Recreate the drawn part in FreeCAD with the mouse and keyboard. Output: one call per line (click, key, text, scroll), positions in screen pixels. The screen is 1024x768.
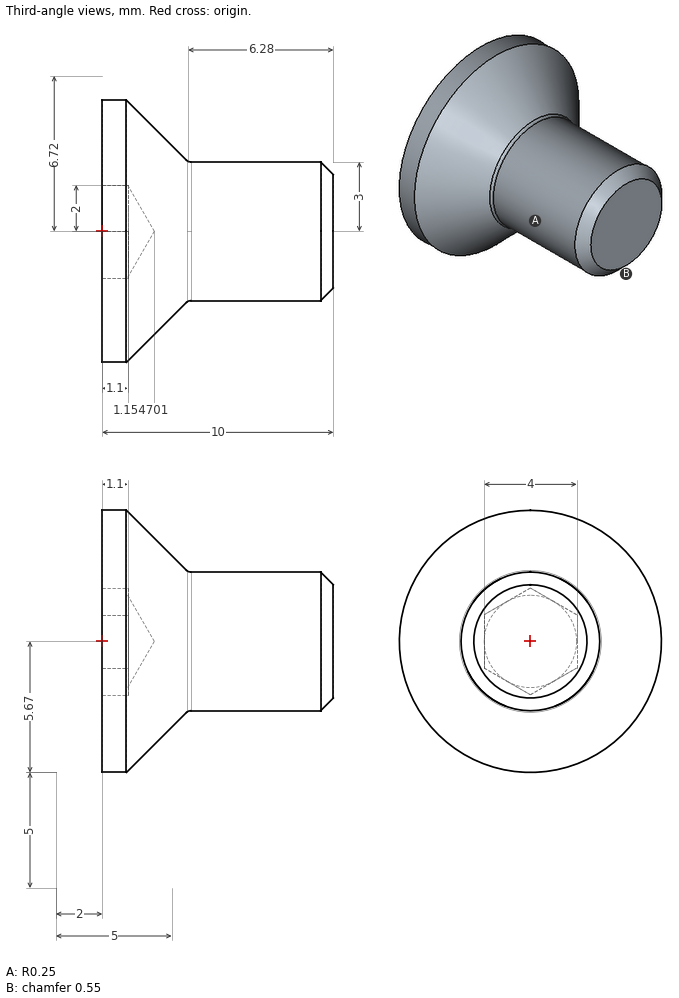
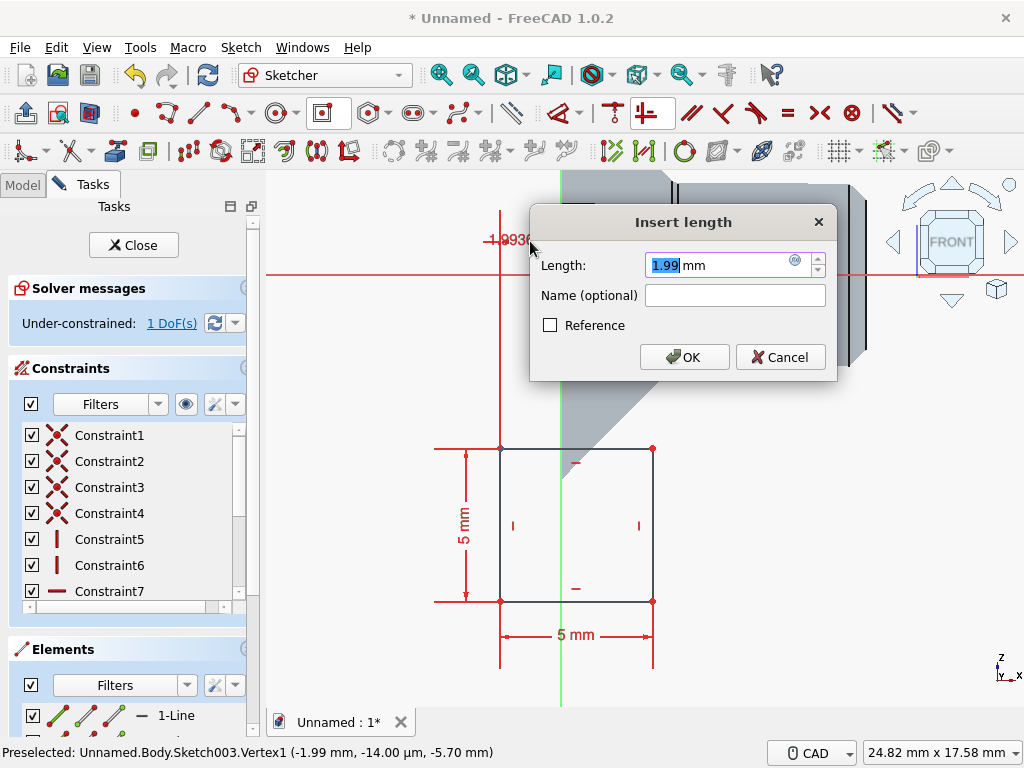
text(2)
key(Return)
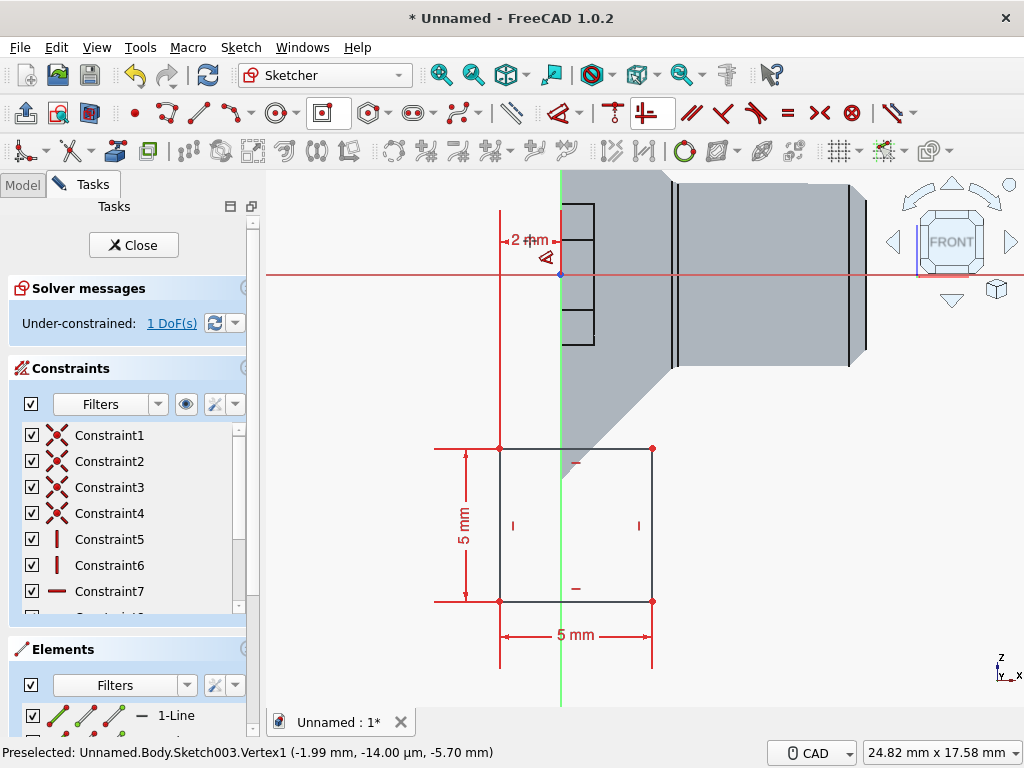
click(500, 449)
click(466, 362)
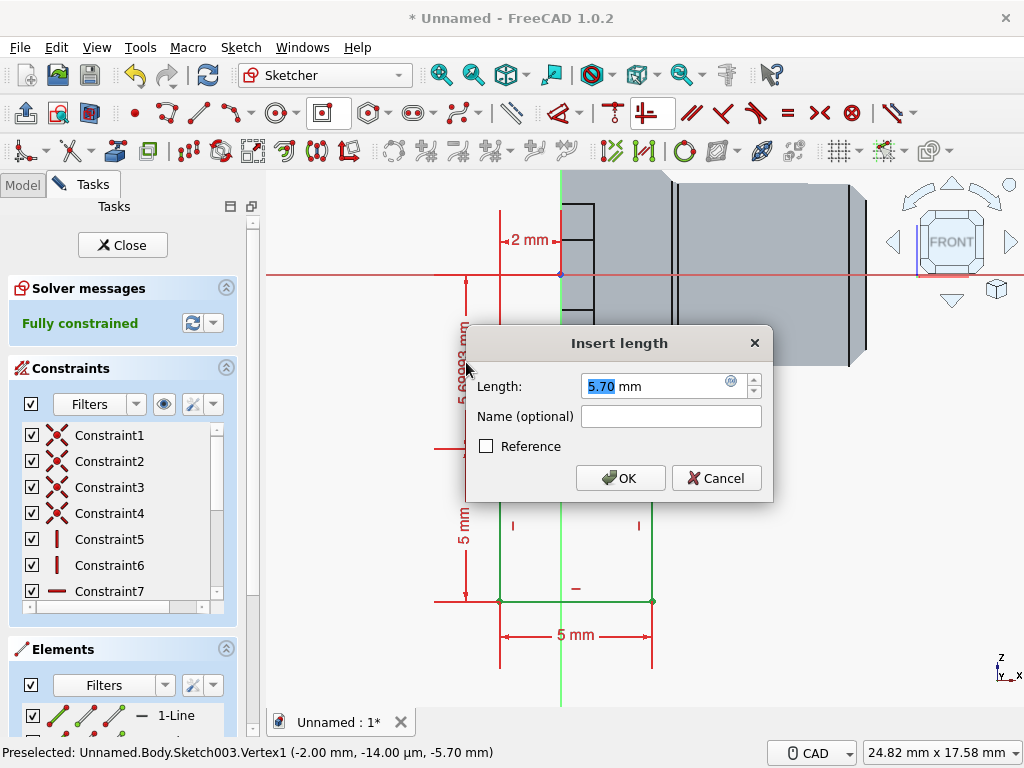
text(5.67)
key(Return)
key(Escape)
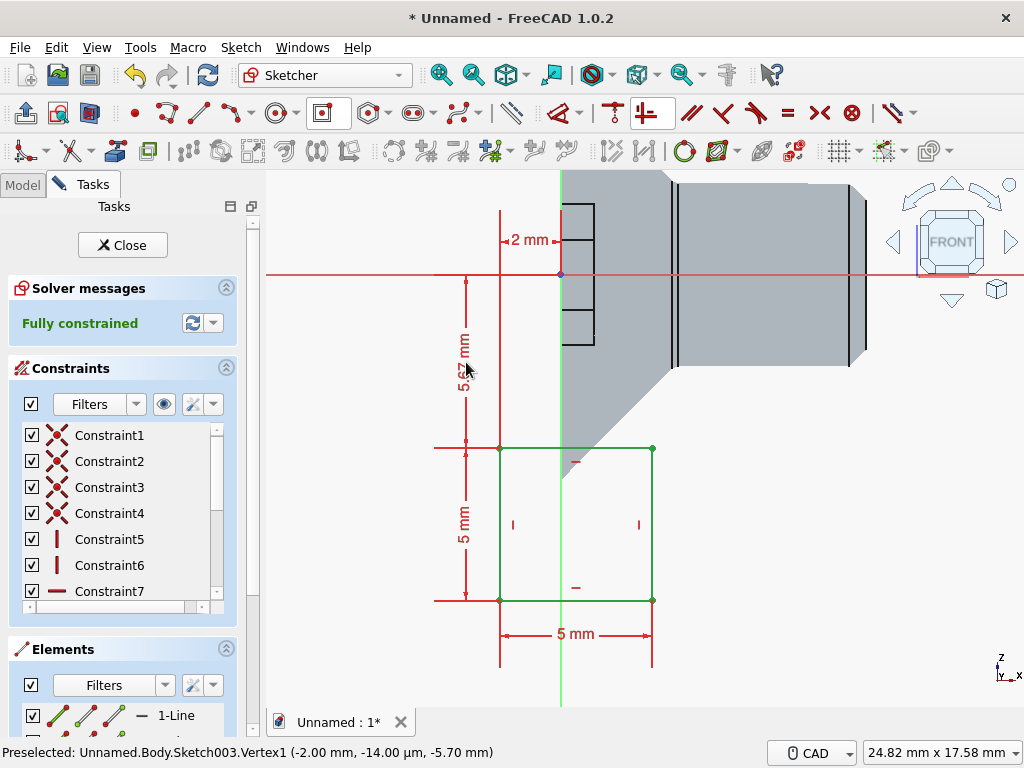
click(123, 245)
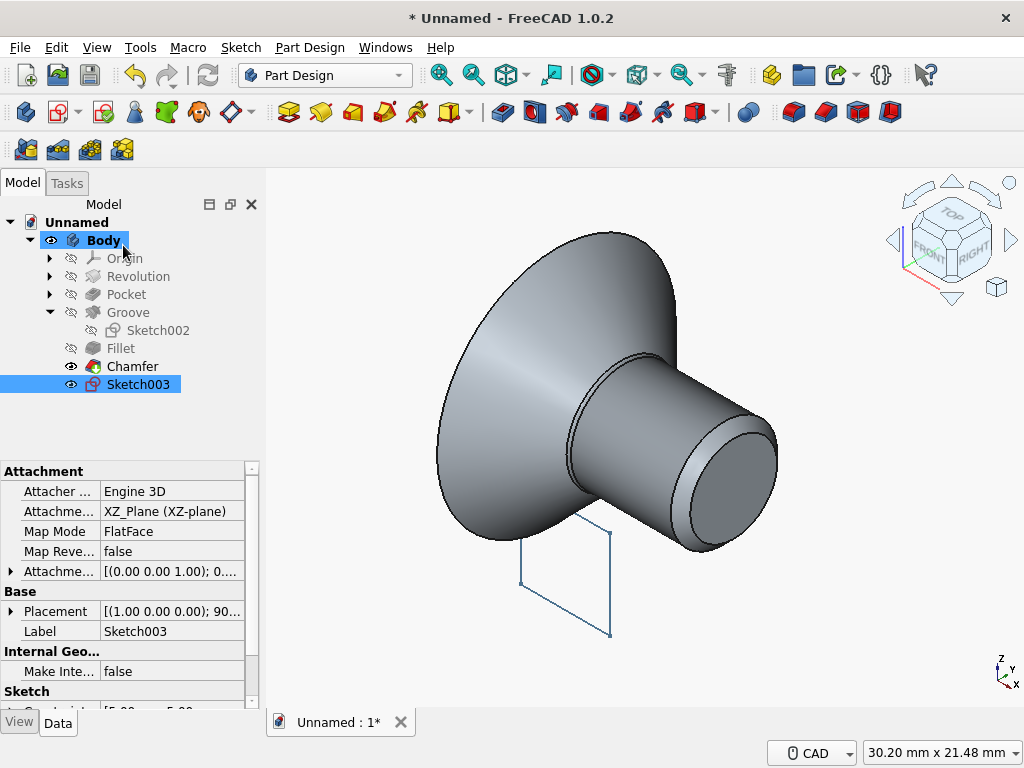
click(568, 112)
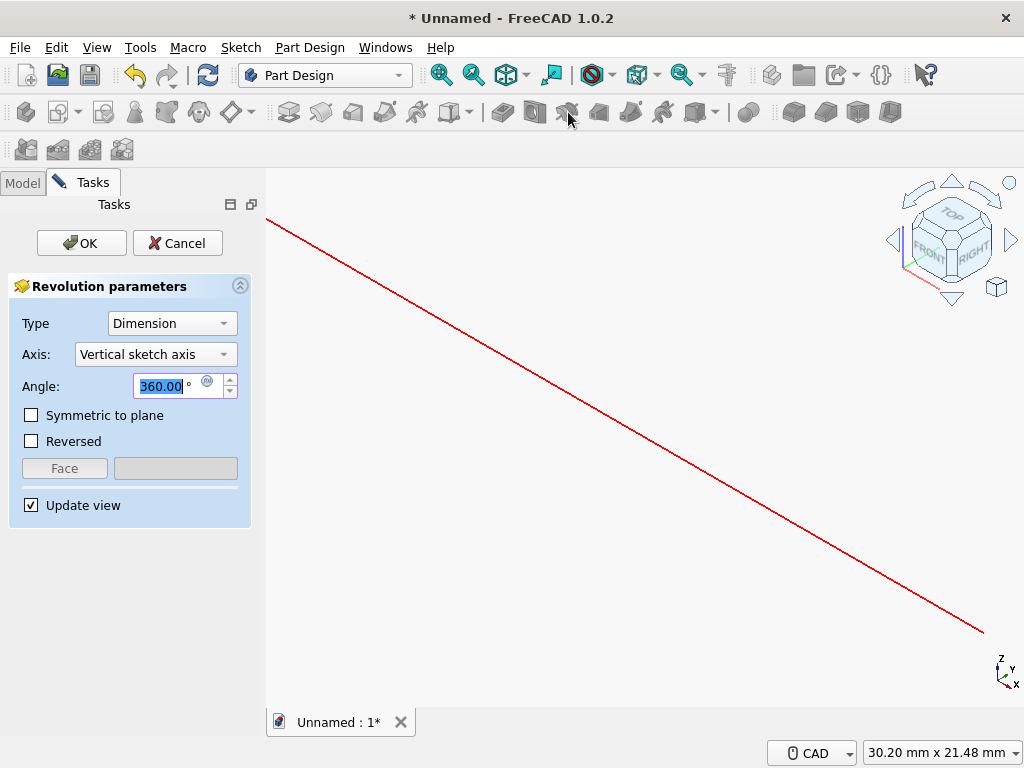
click(156, 354)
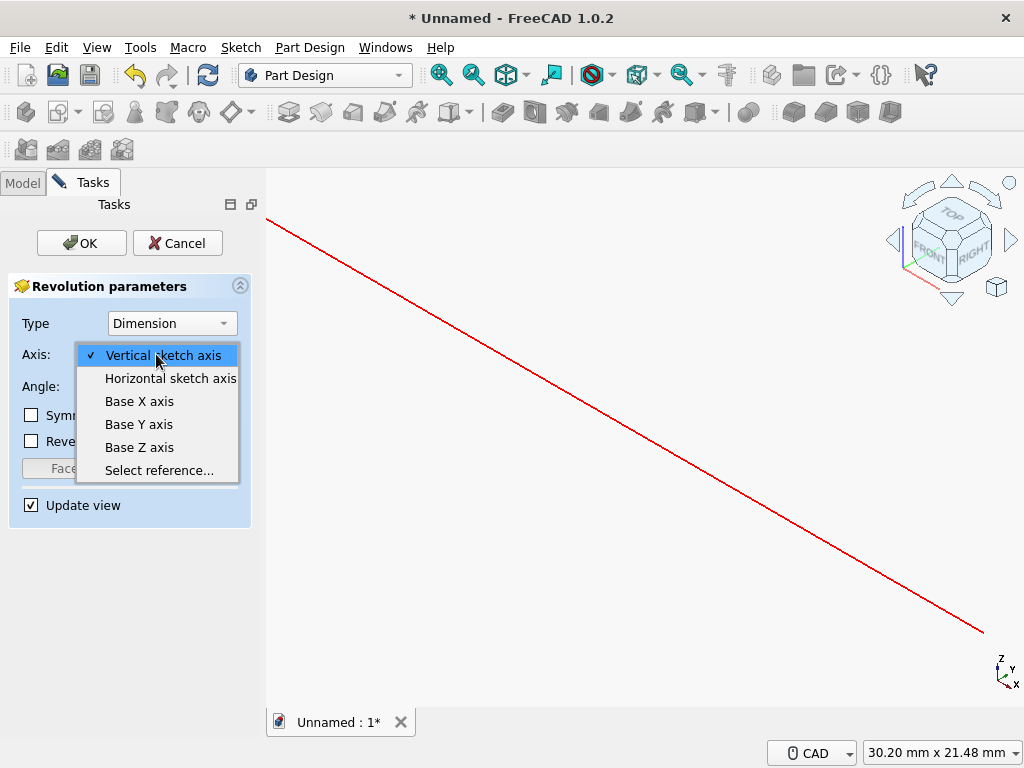
click(156, 378)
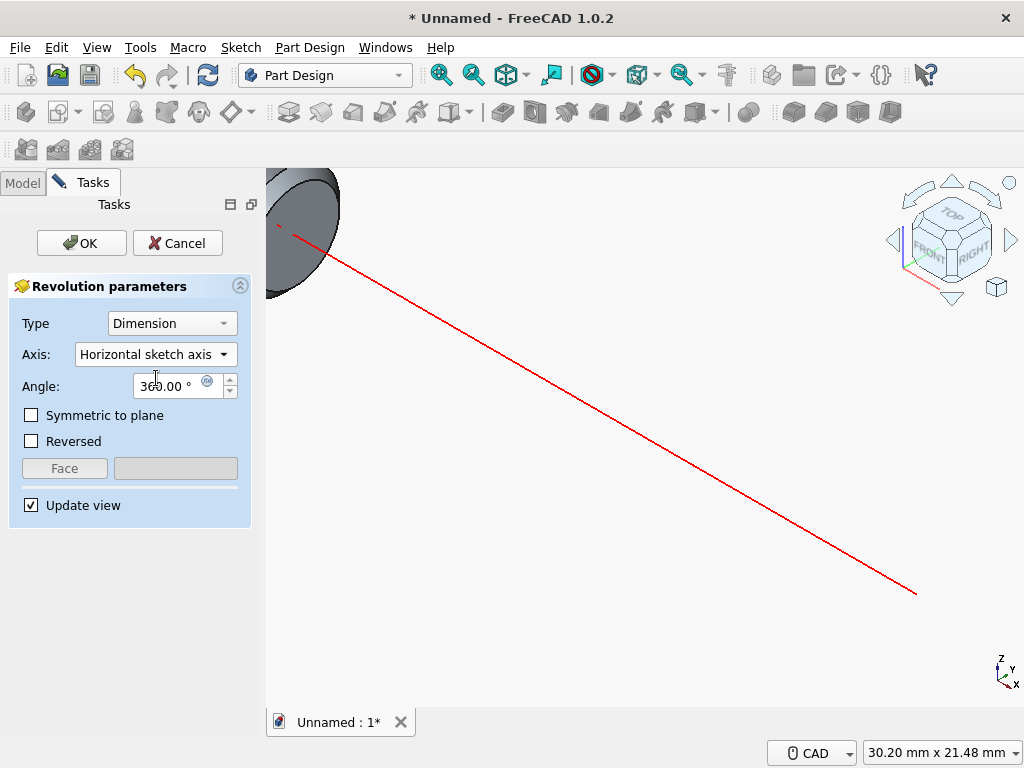
click(82, 243)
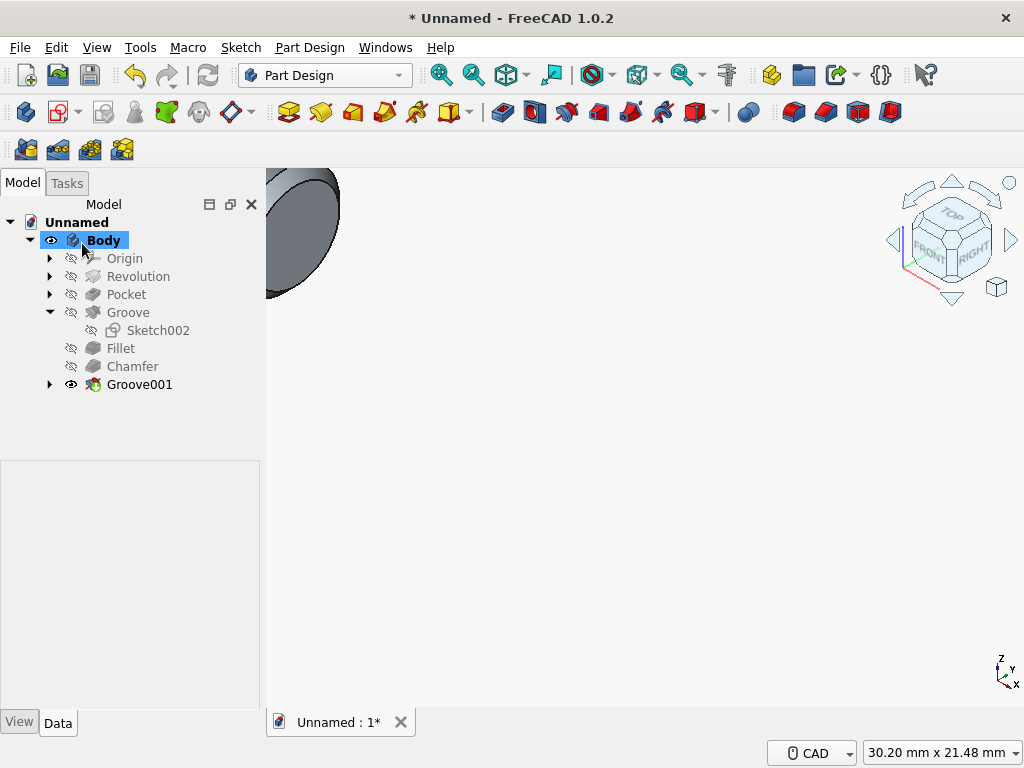
key(v)
key(f)